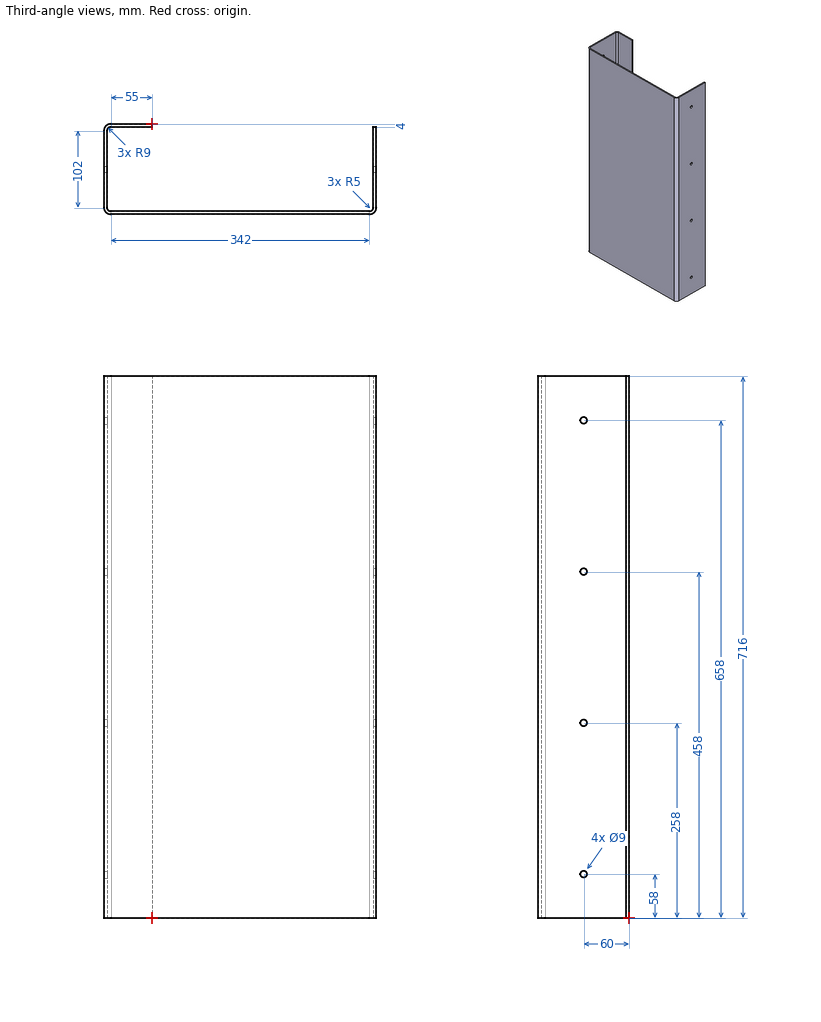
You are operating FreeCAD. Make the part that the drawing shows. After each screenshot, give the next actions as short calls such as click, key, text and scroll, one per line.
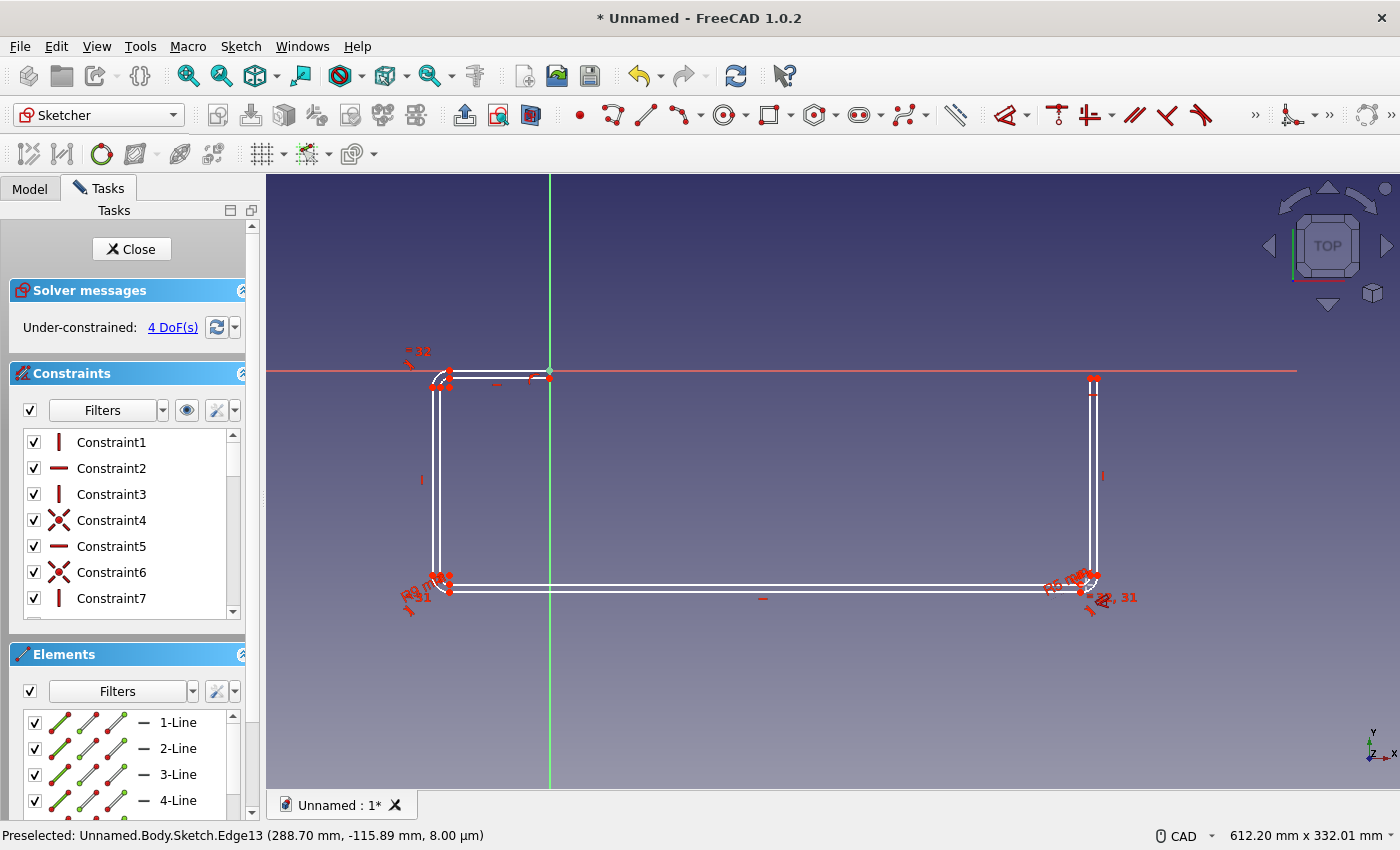
scroll(480, 378, up, 4)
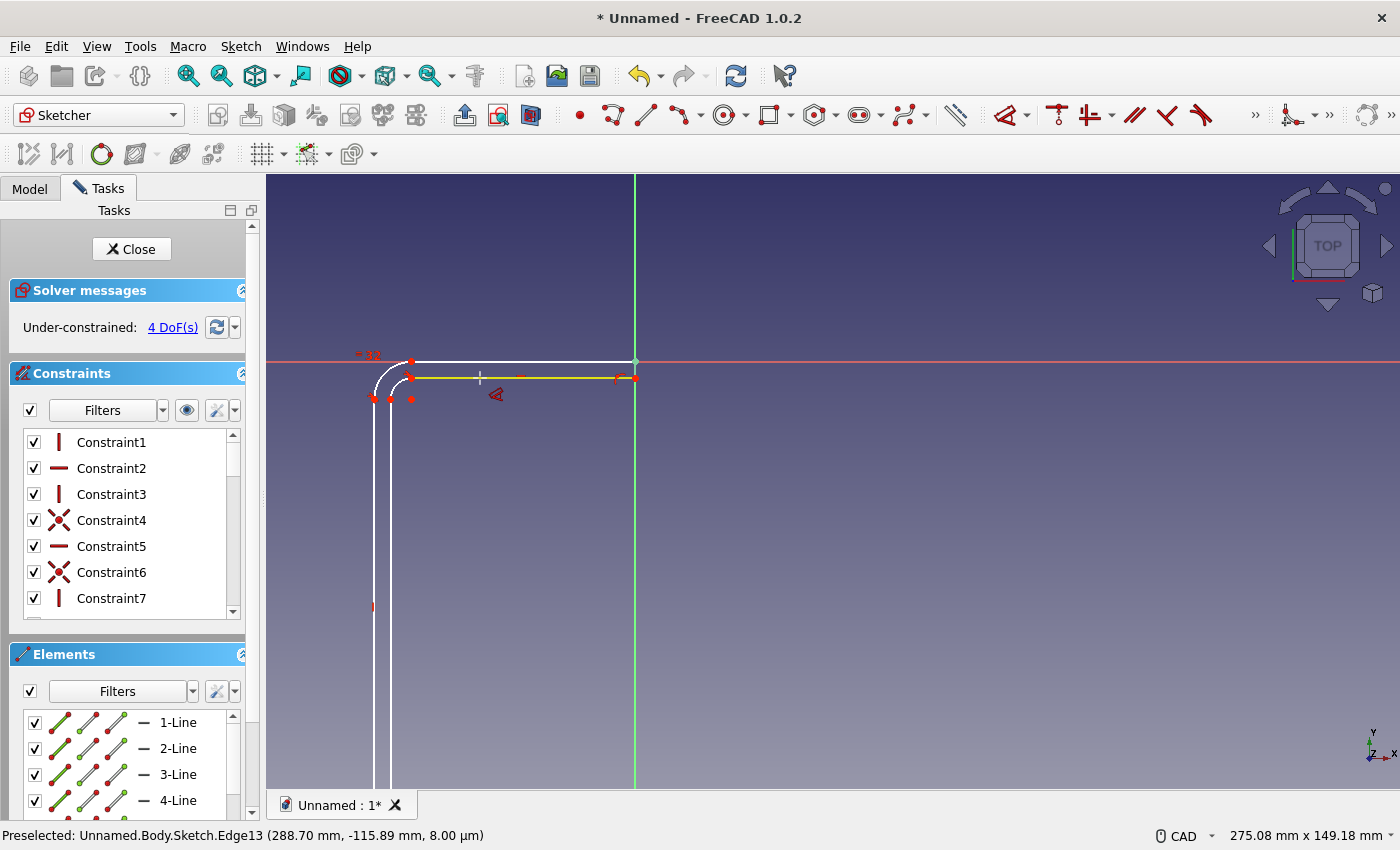
click(479, 378)
click(524, 344)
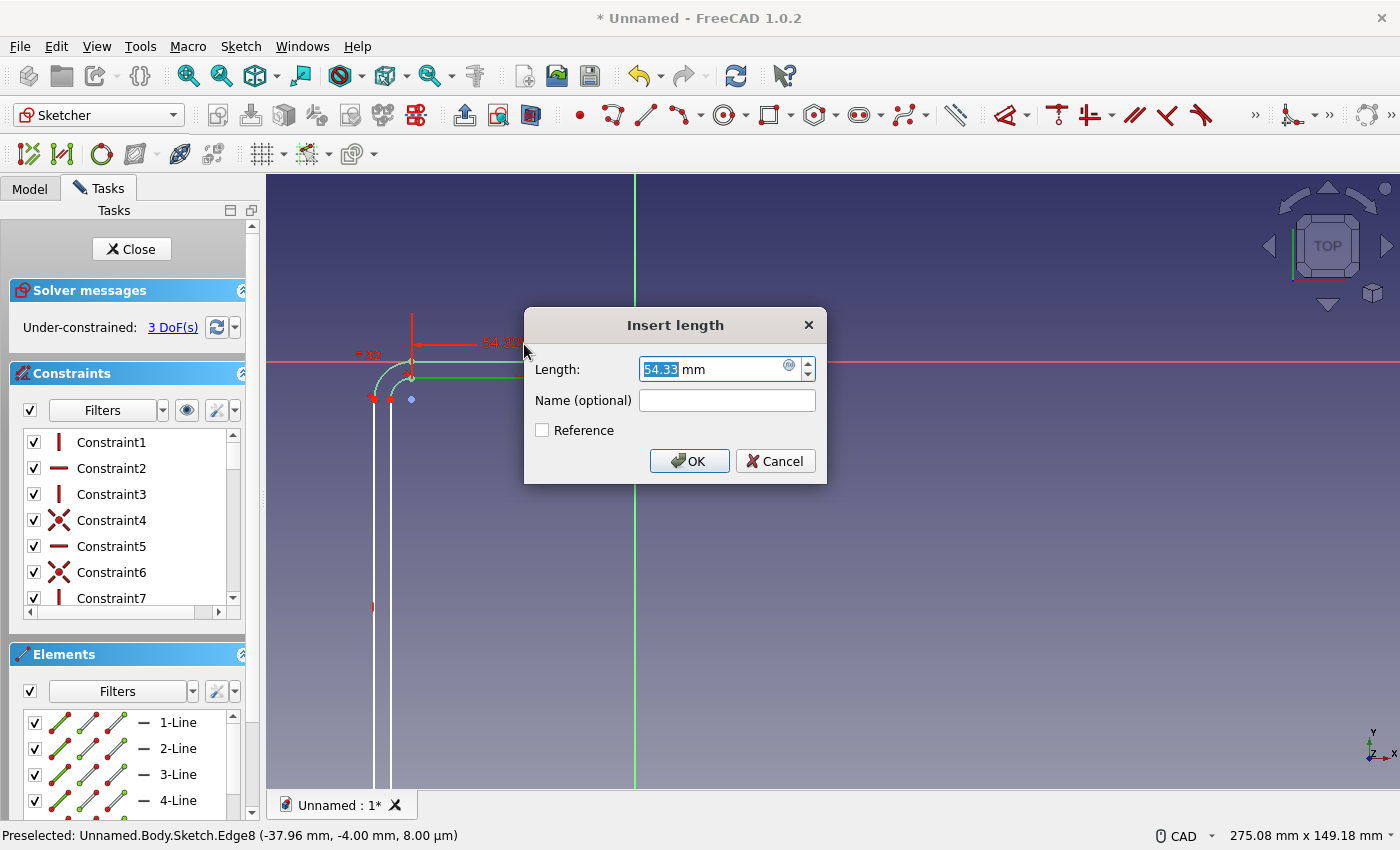
text(55)
key(Return)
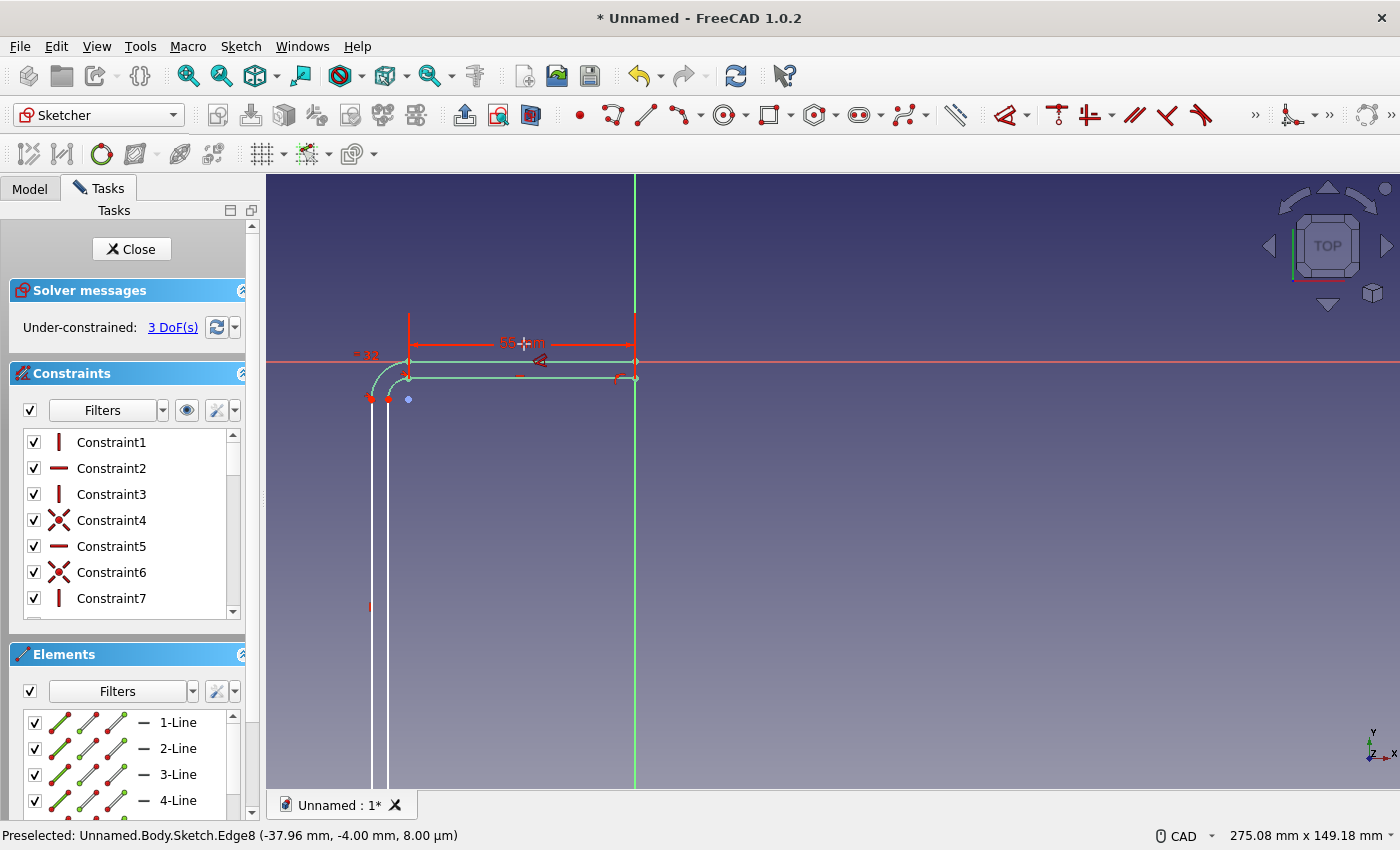
scroll(480, 377, down, 4)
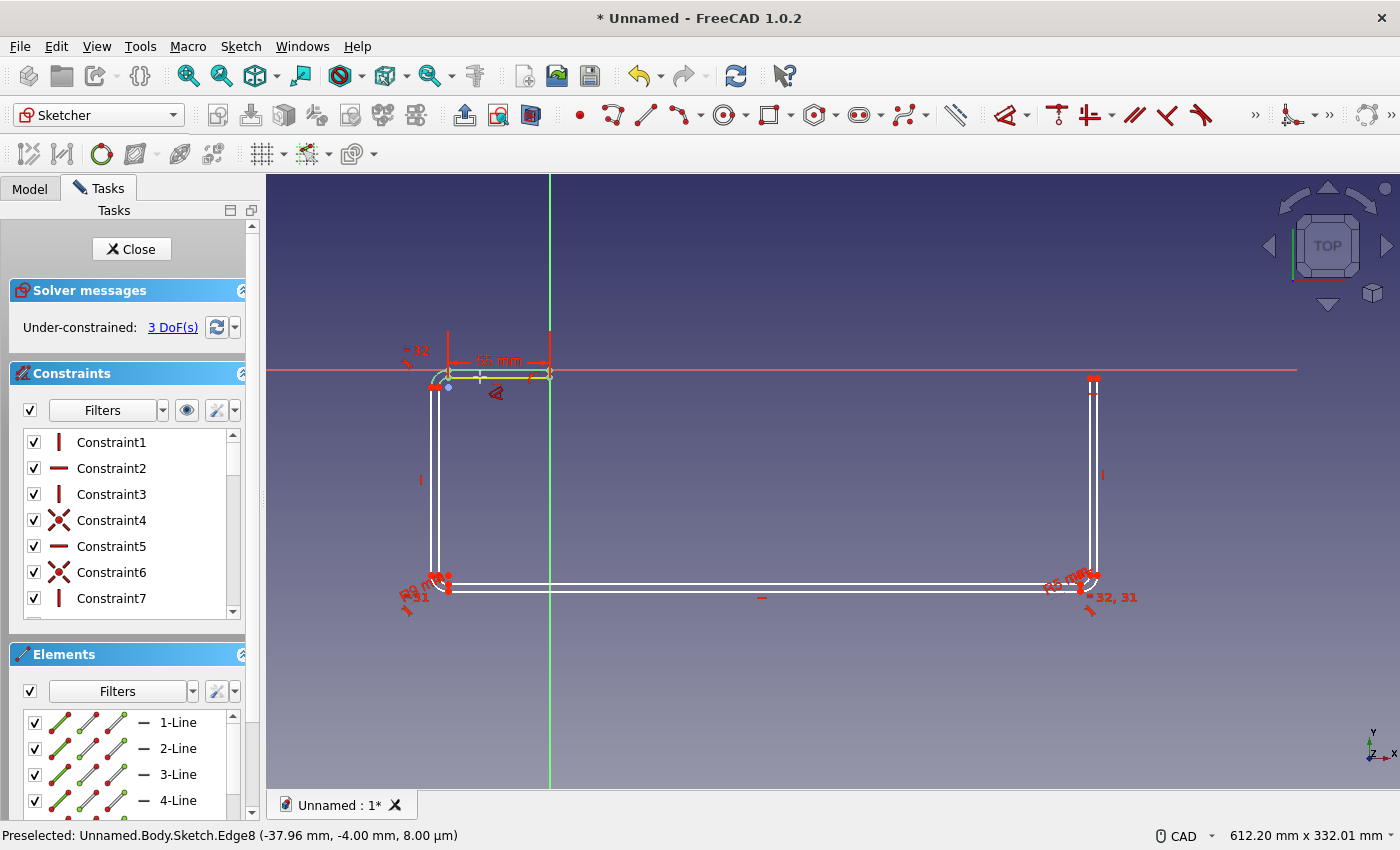
scroll(1097, 378, up, 9)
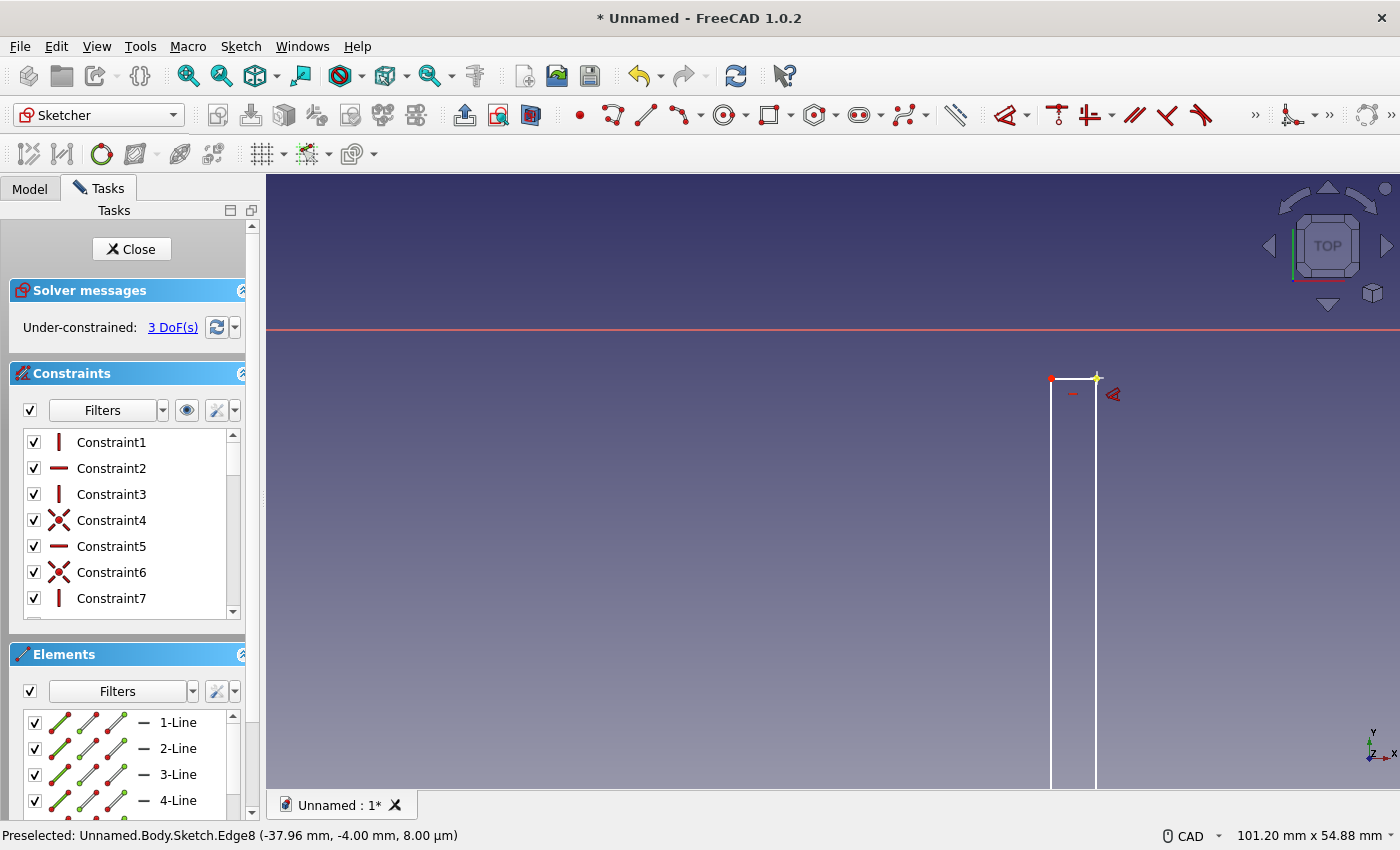
click(1096, 379)
click(1130, 354)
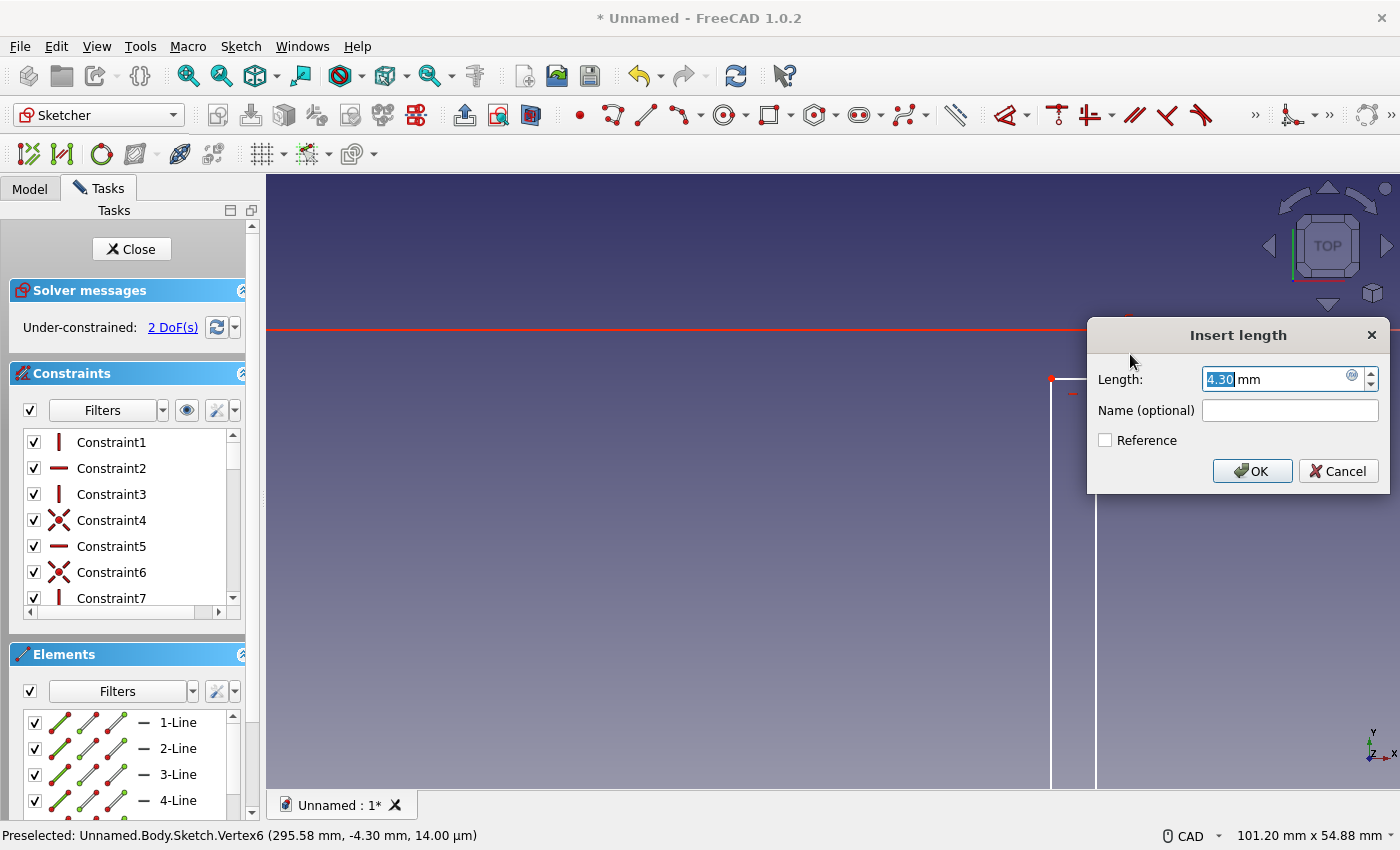
text(4)
key(Return)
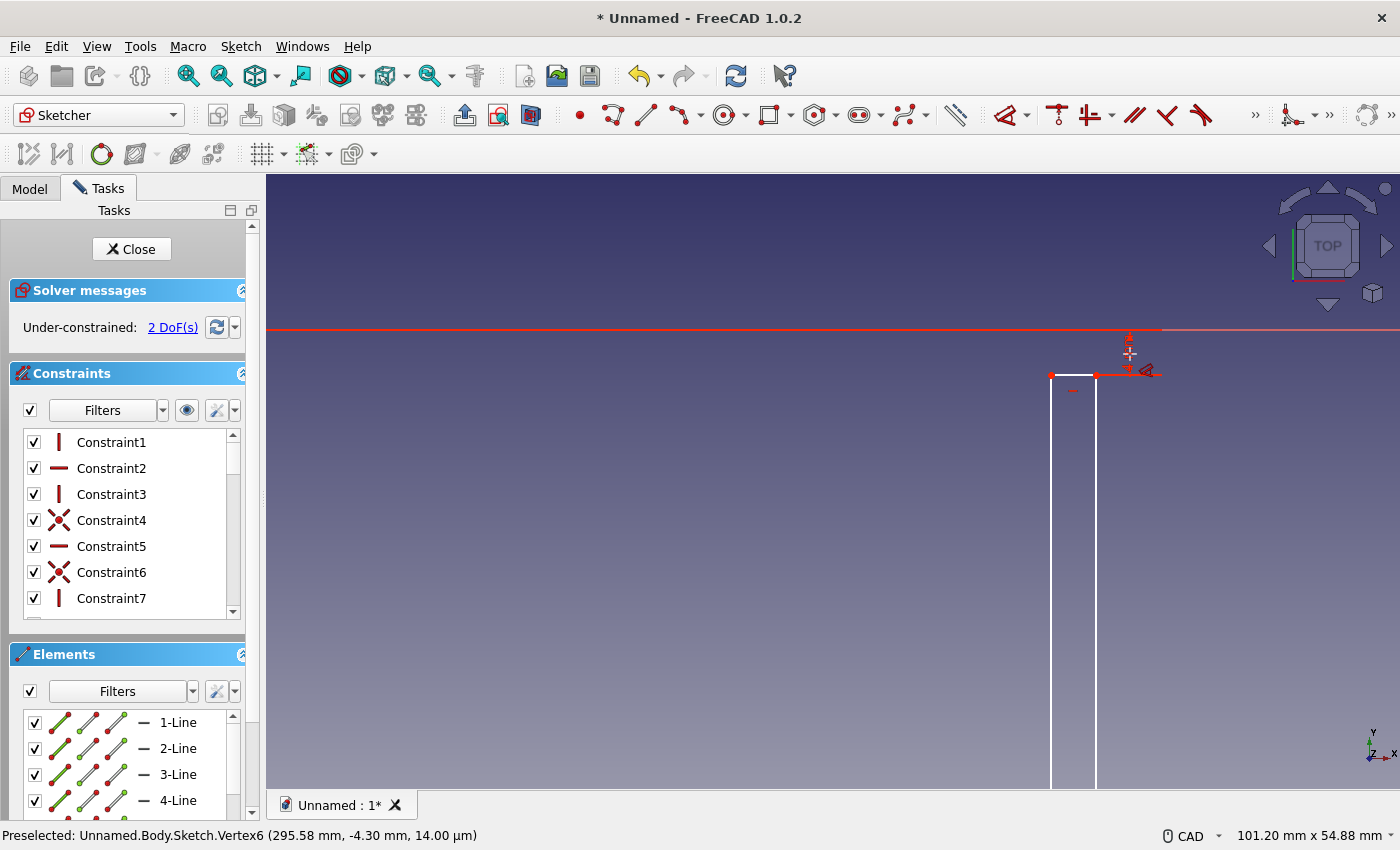
scroll(1097, 378, down, 9)